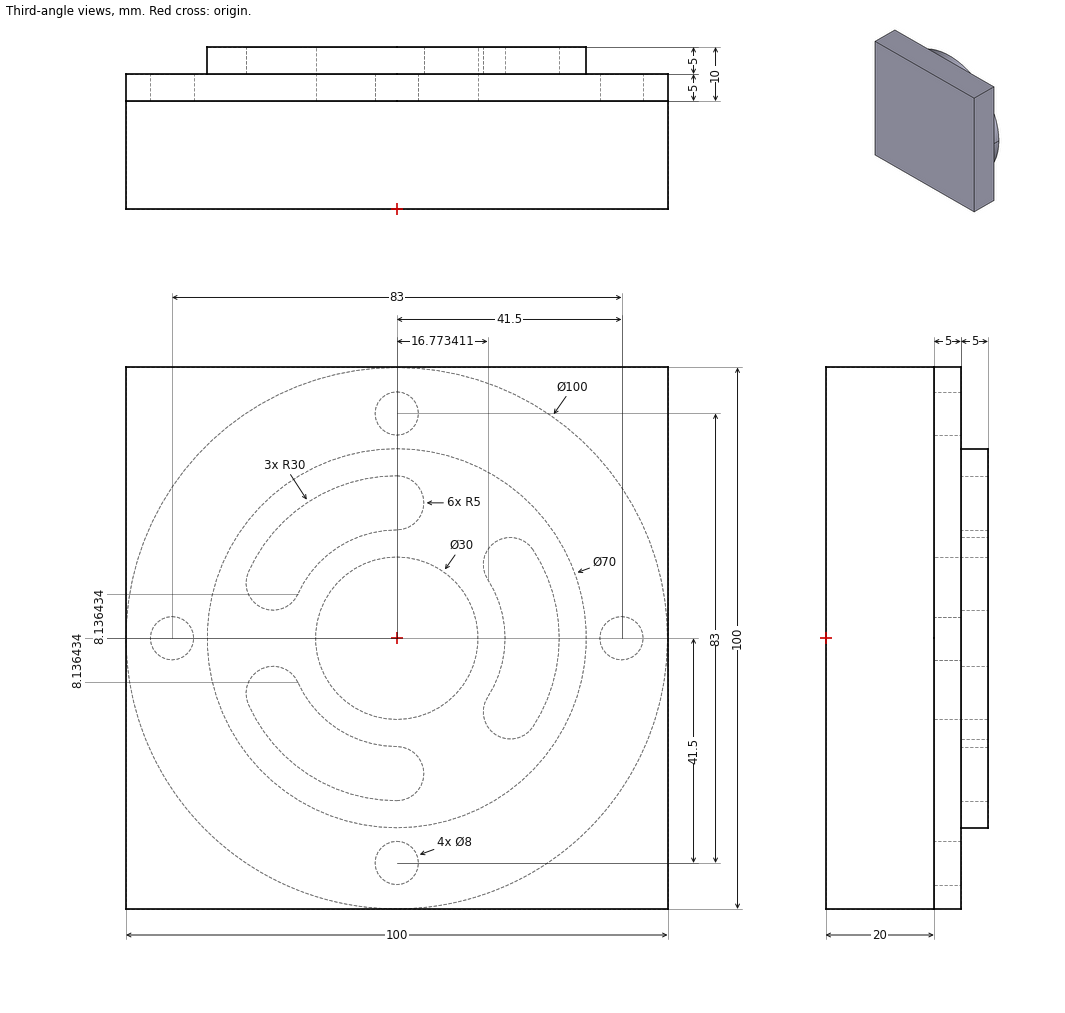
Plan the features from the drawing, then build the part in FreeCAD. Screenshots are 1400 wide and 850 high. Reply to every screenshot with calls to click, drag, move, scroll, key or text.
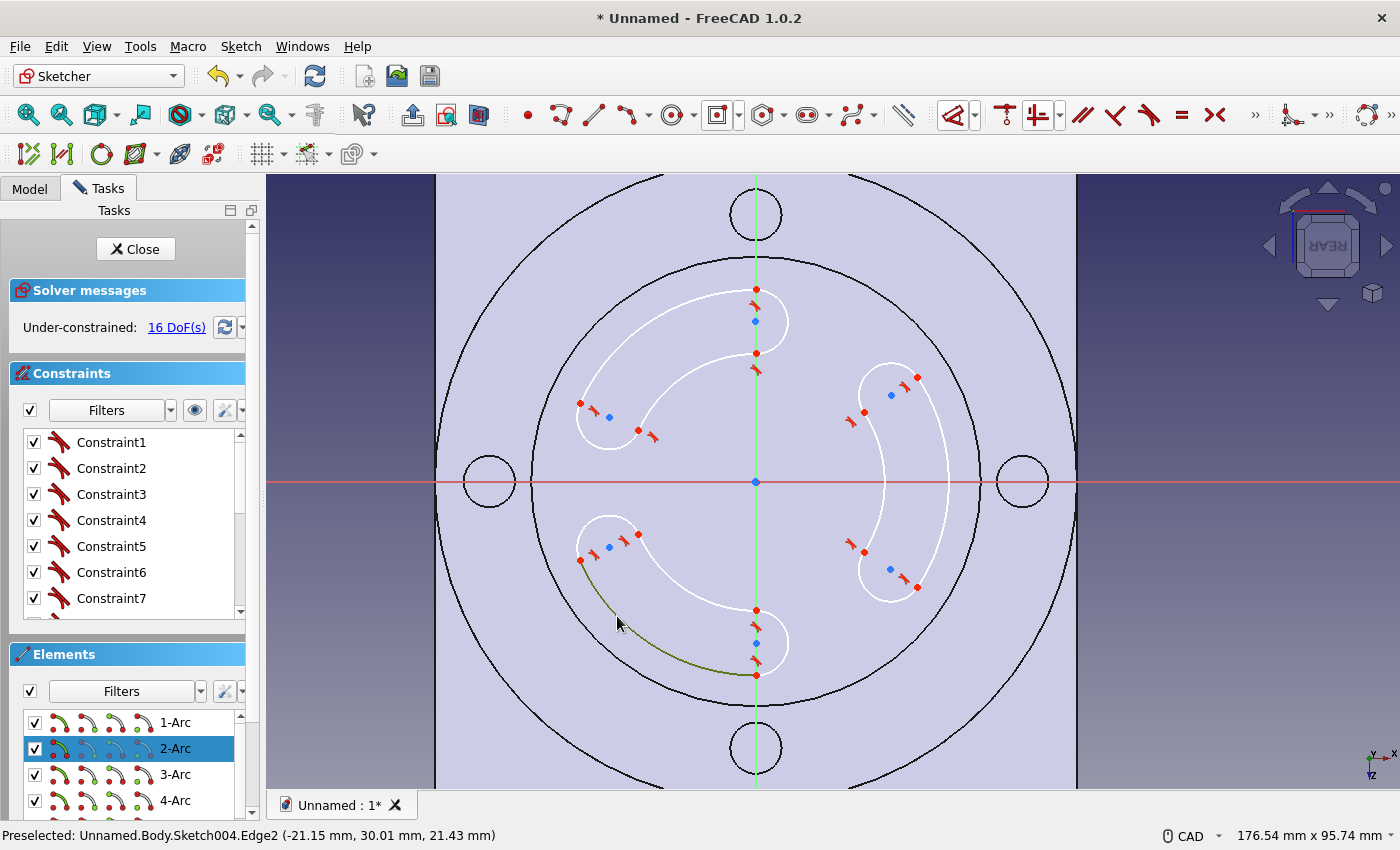
click(691, 301)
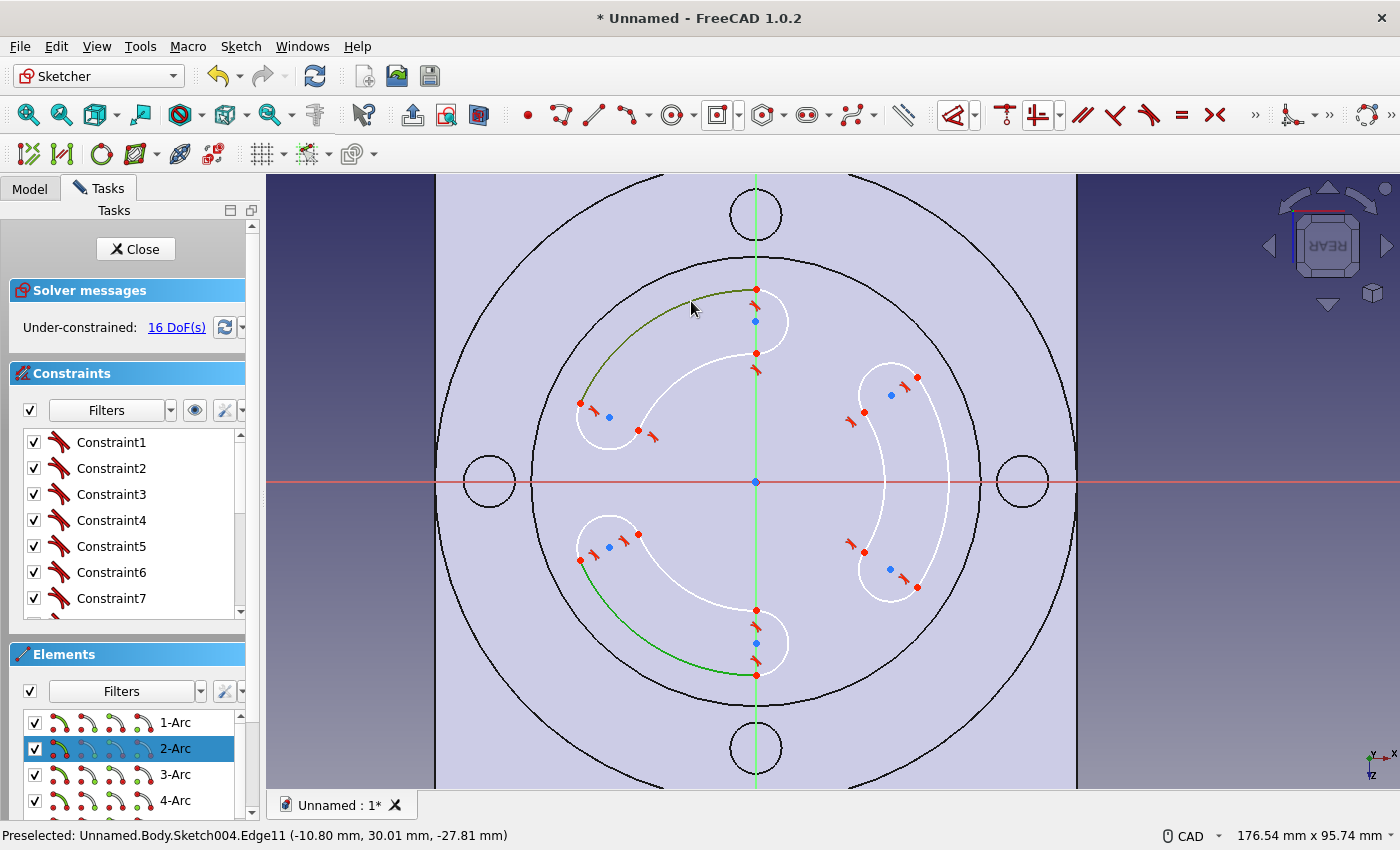
click(1005, 116)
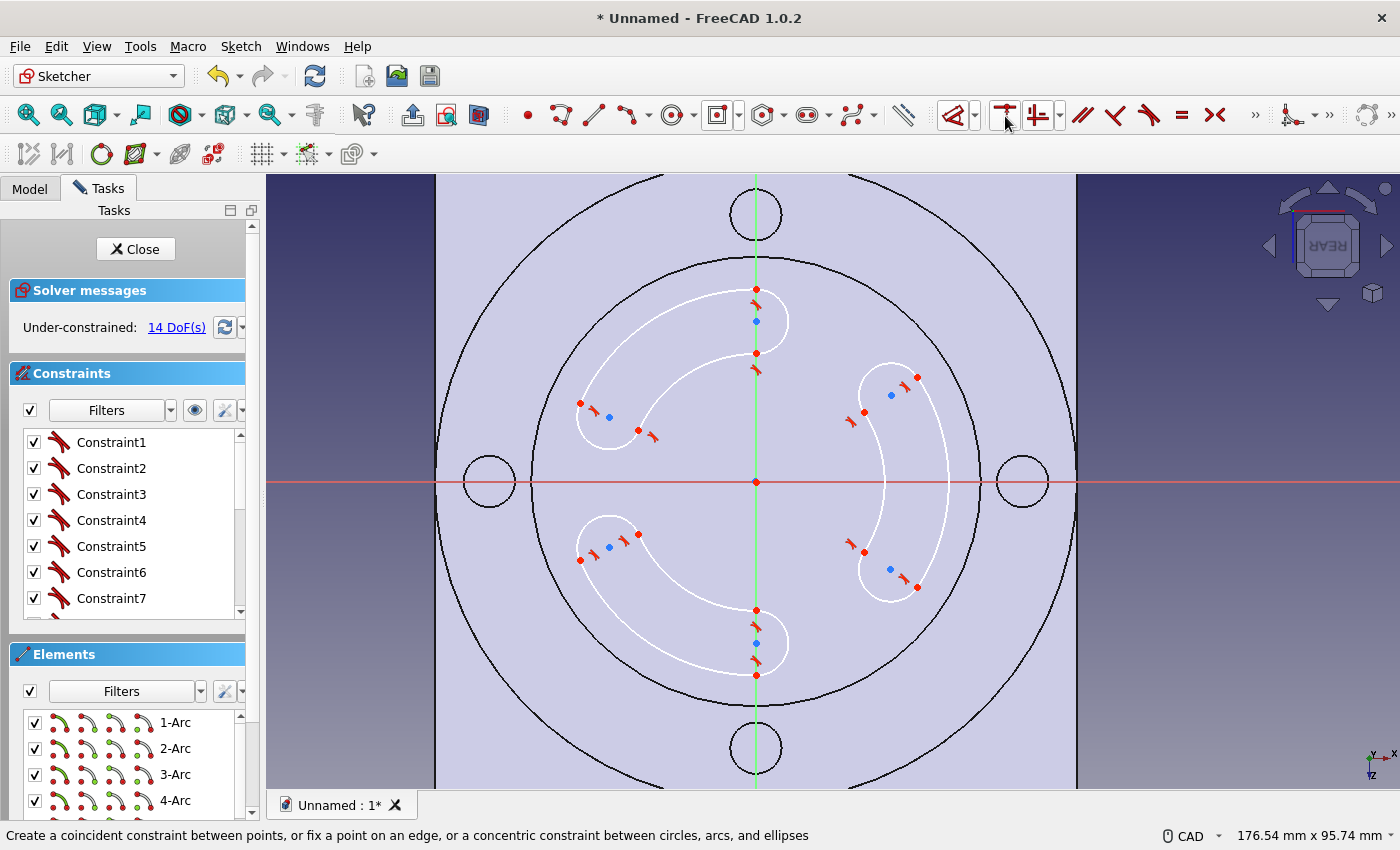
scroll(756, 482, up, 2)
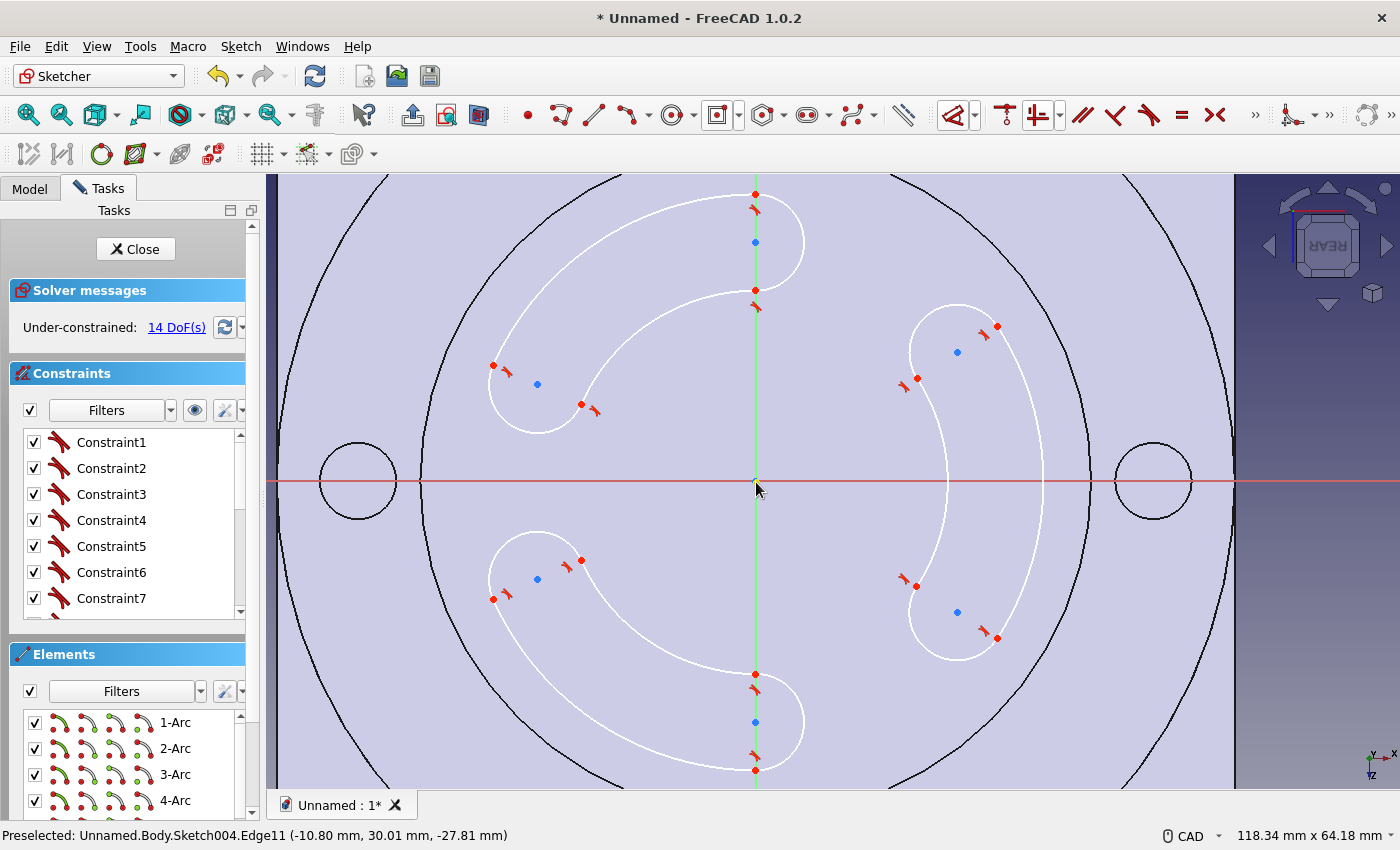
drag(746, 471, 766, 492)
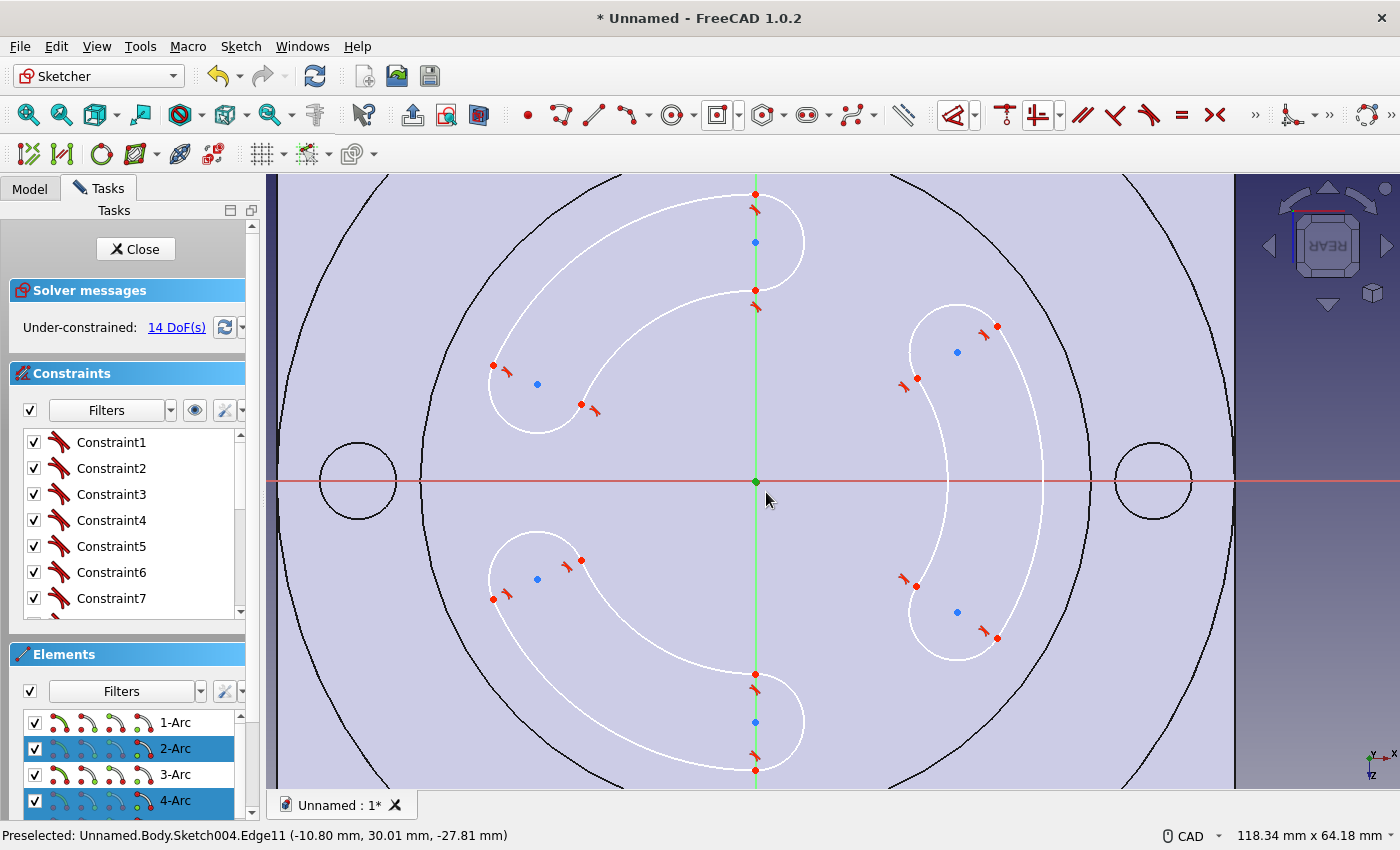
click(1005, 116)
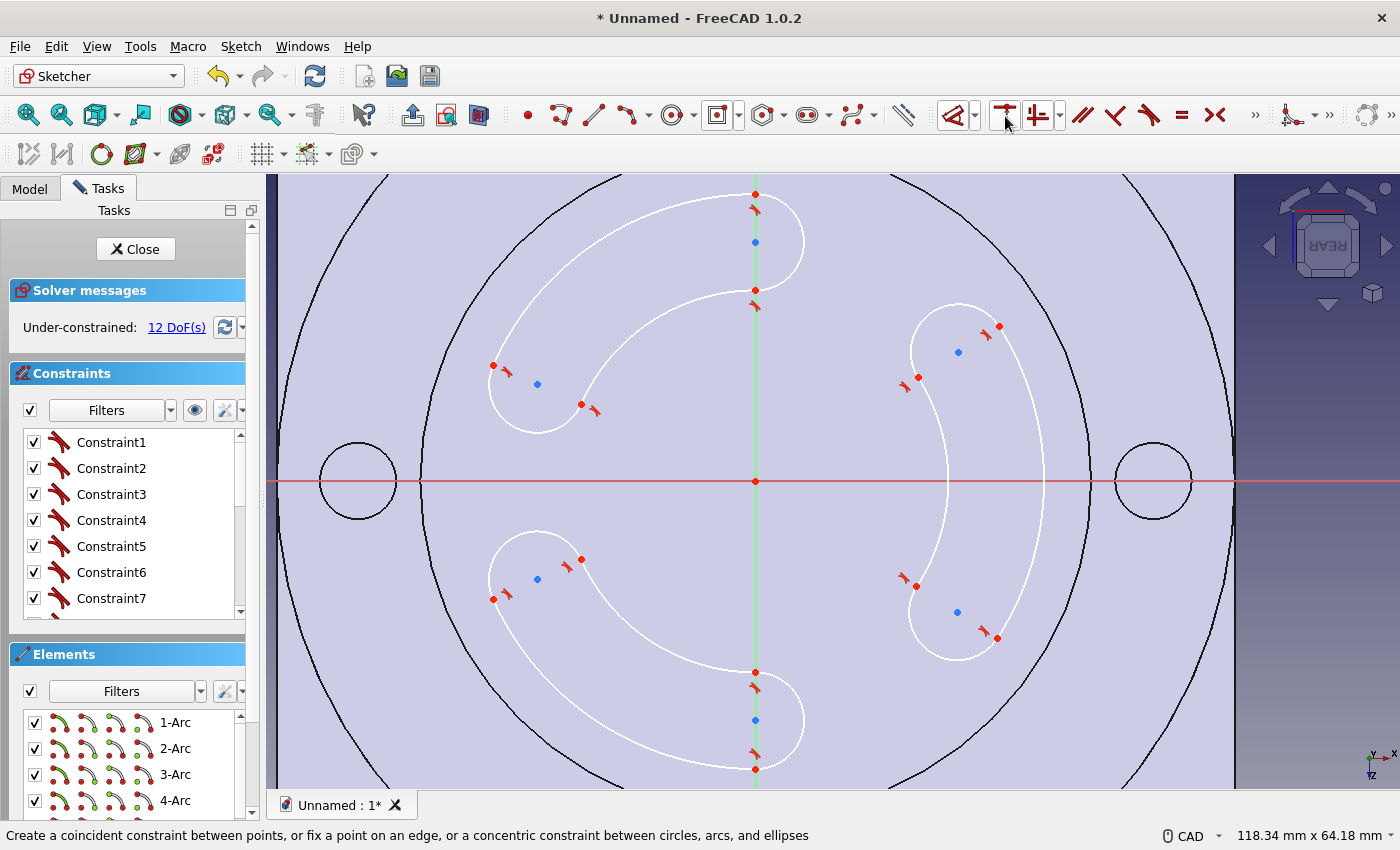
click(618, 614)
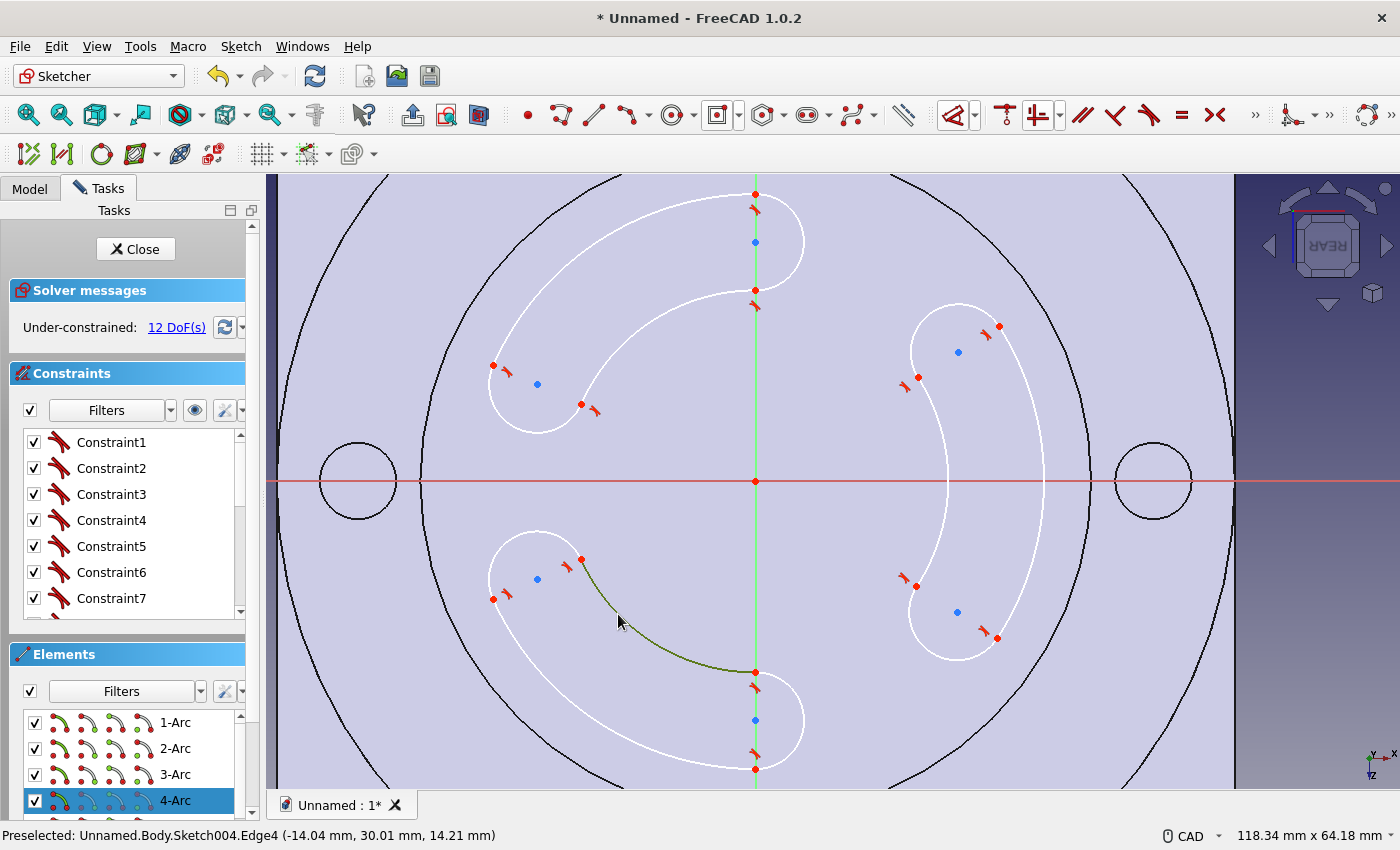
click(943, 526)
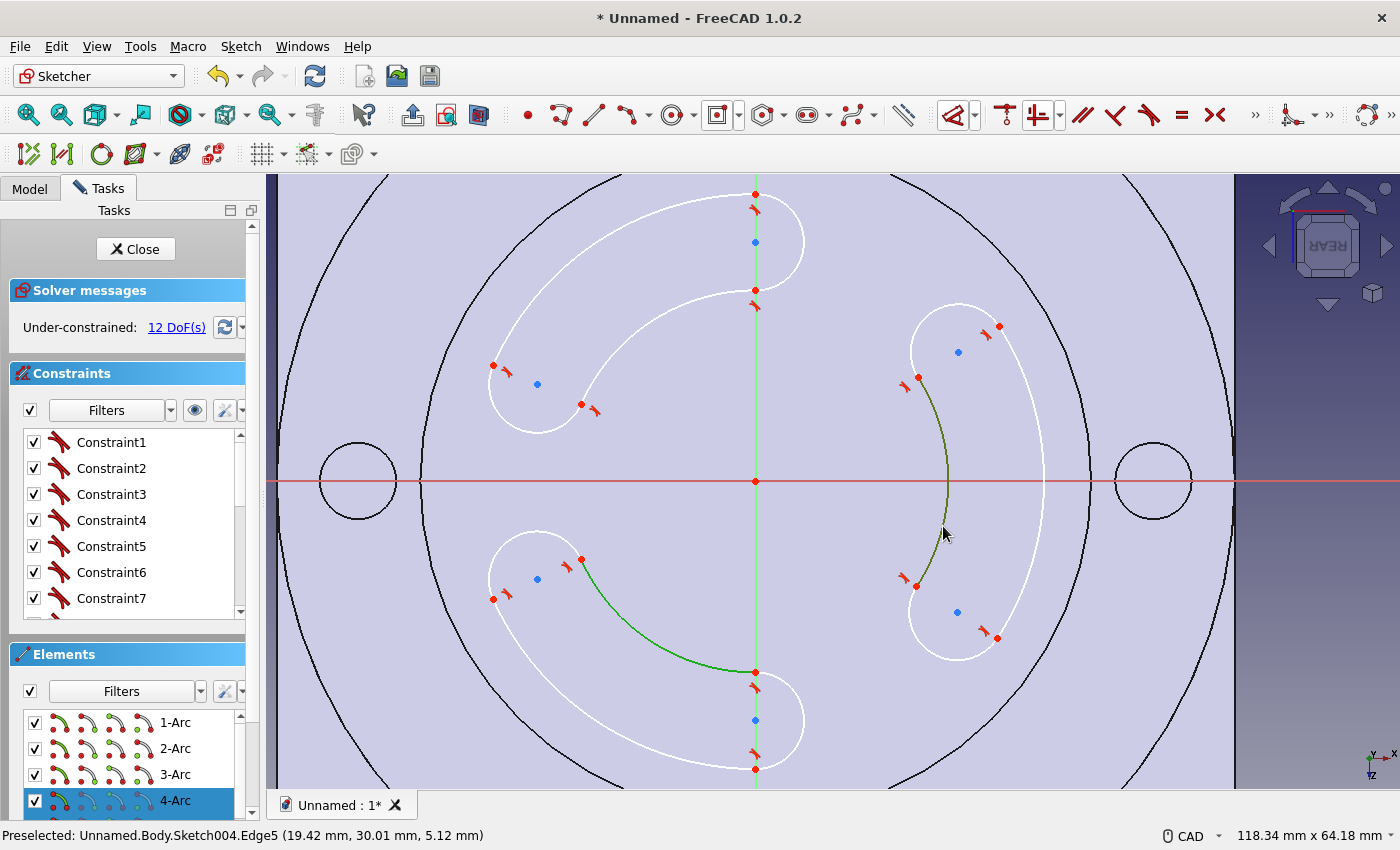
click(691, 302)